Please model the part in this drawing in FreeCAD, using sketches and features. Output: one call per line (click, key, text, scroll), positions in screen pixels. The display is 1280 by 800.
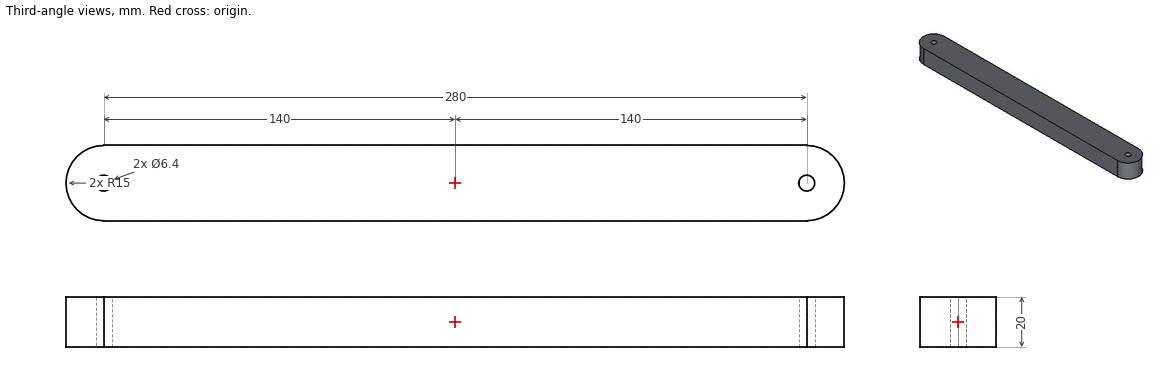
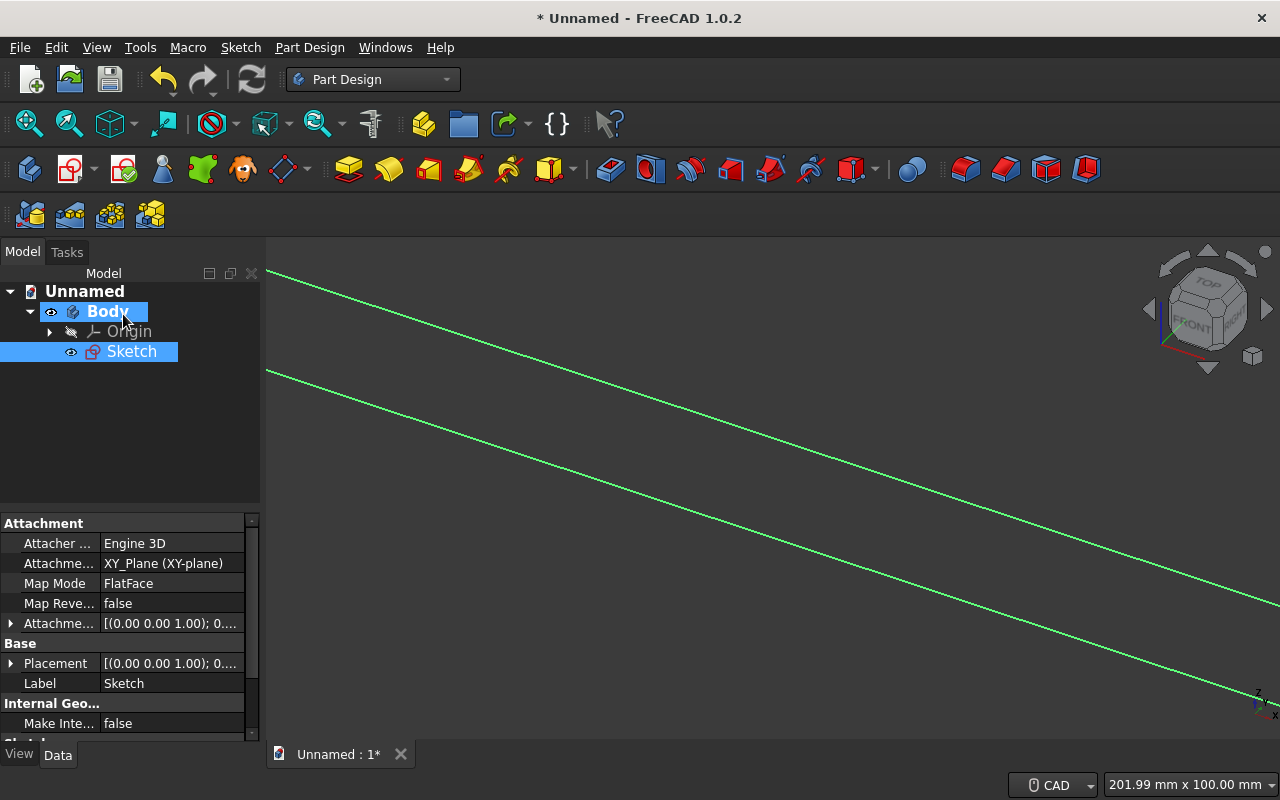
click(350, 170)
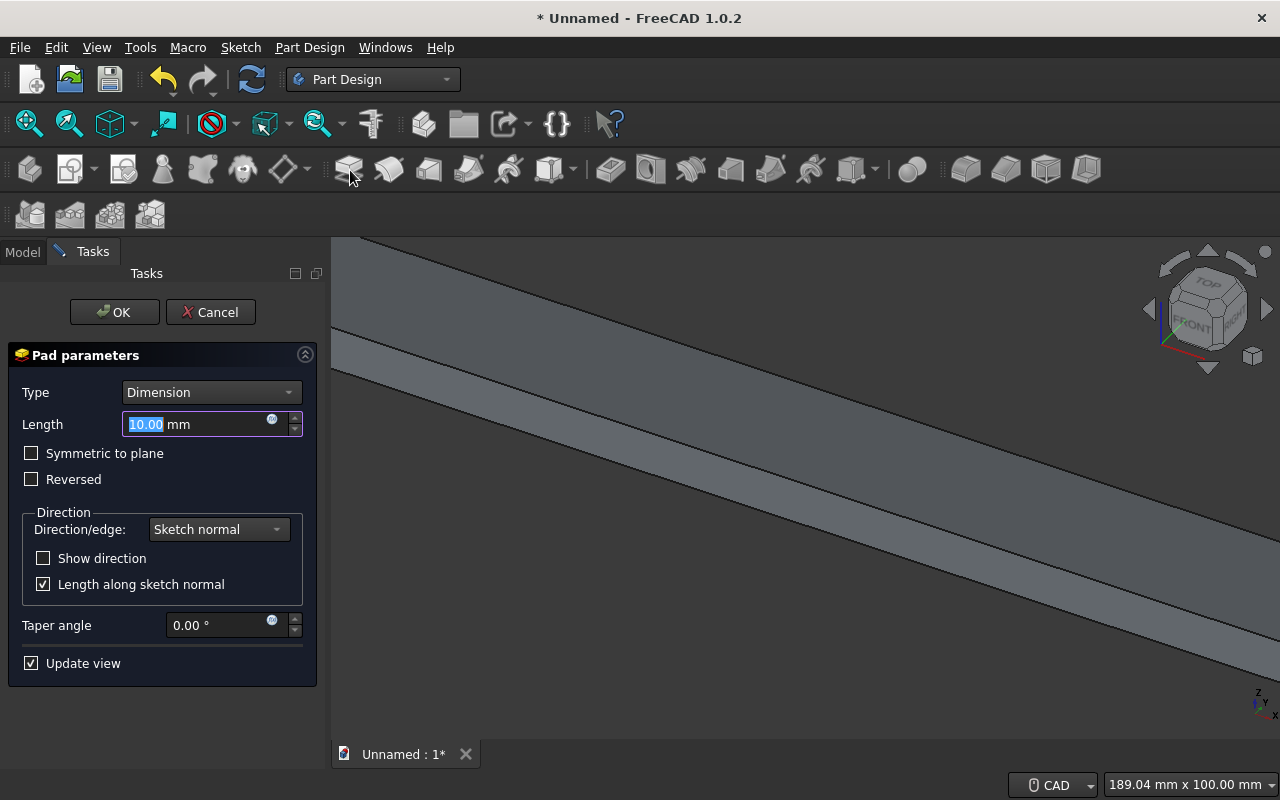
text(20)
key(Tab)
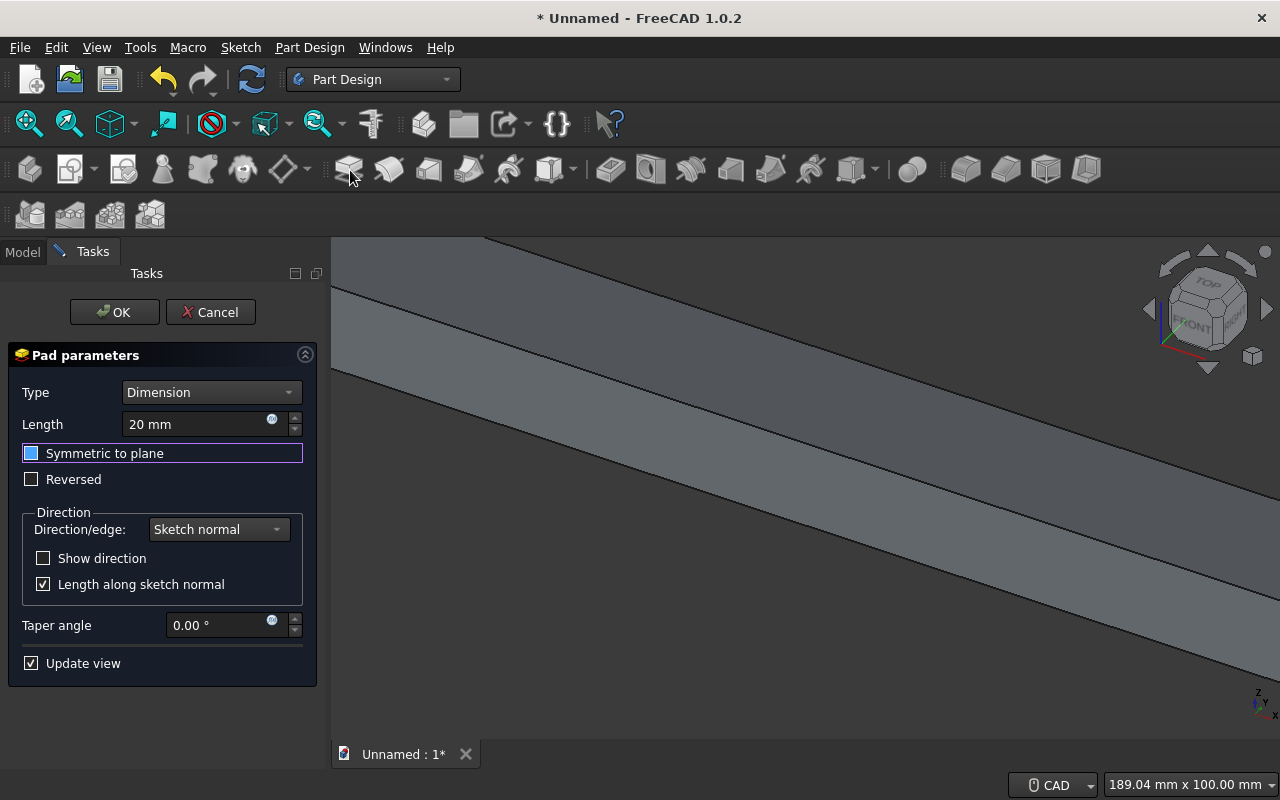
click(30, 453)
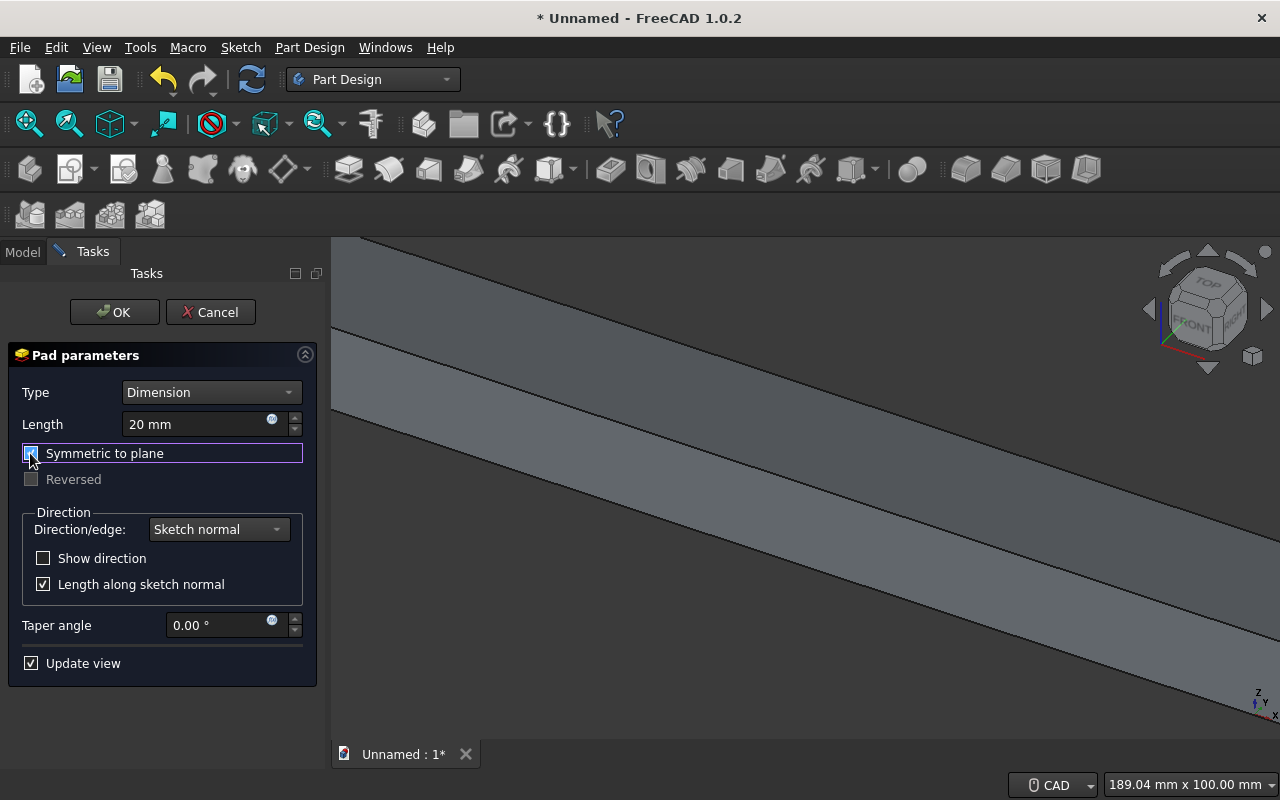
click(115, 312)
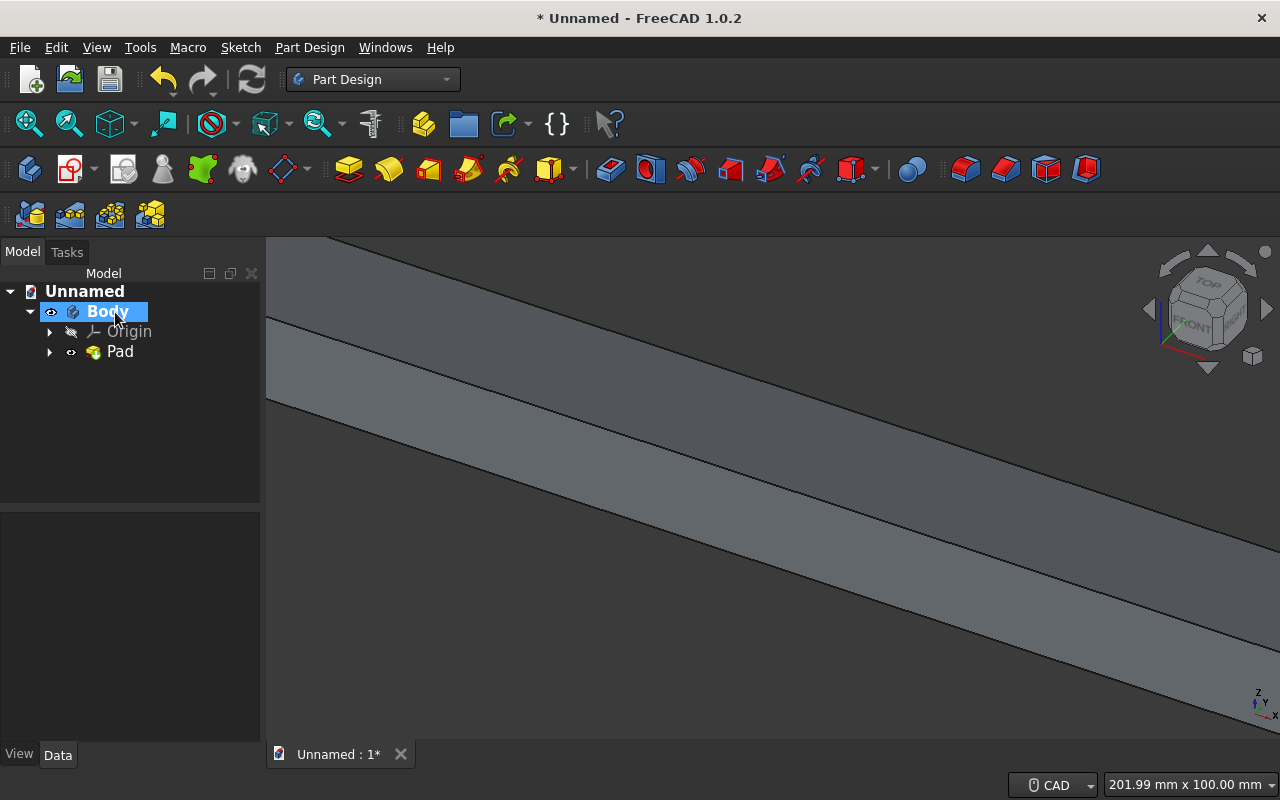
click(30, 124)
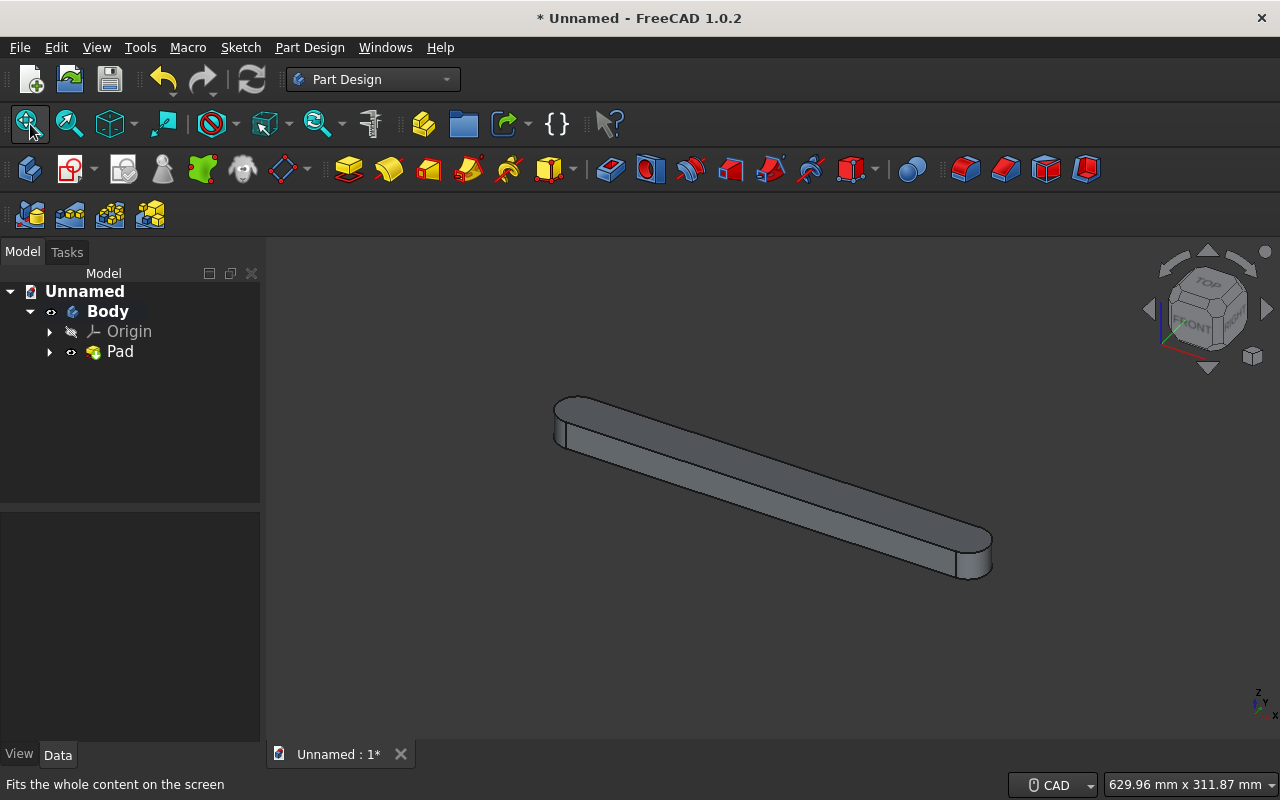
click(70, 170)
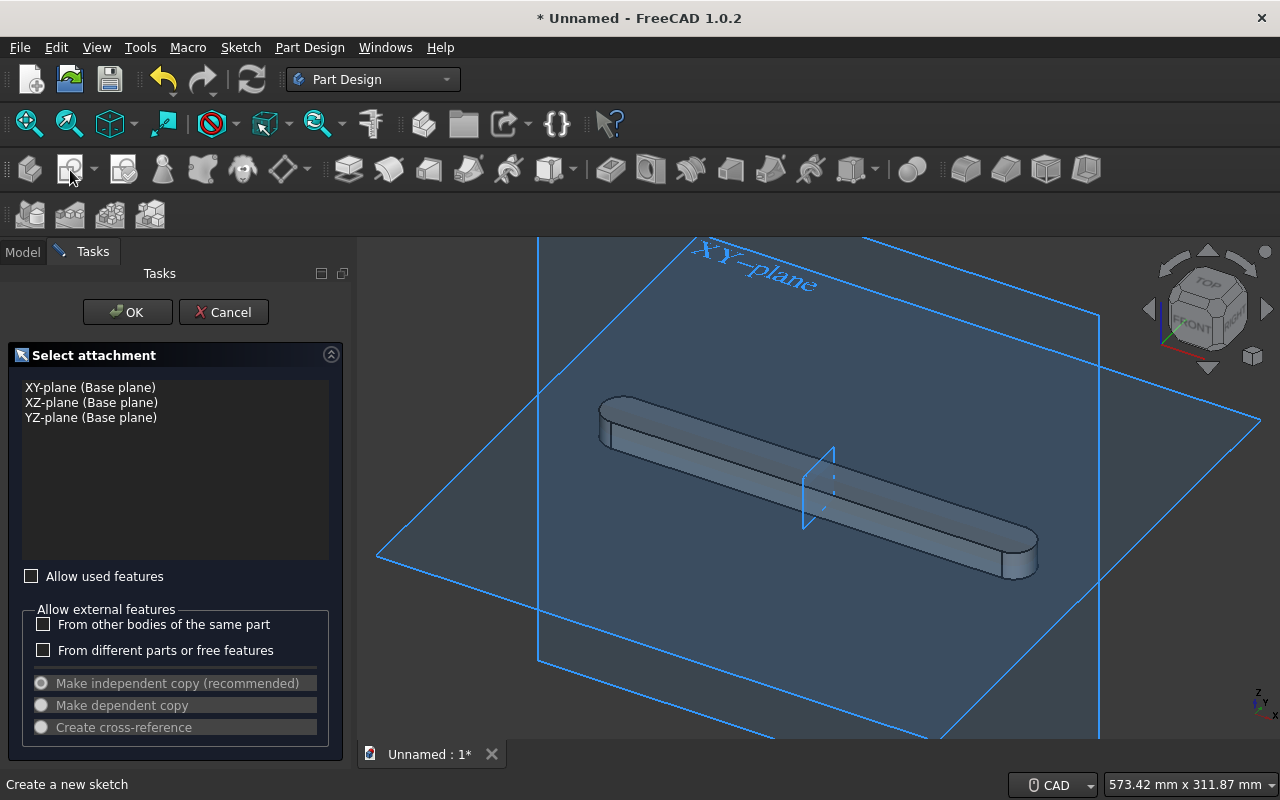
click(82, 388)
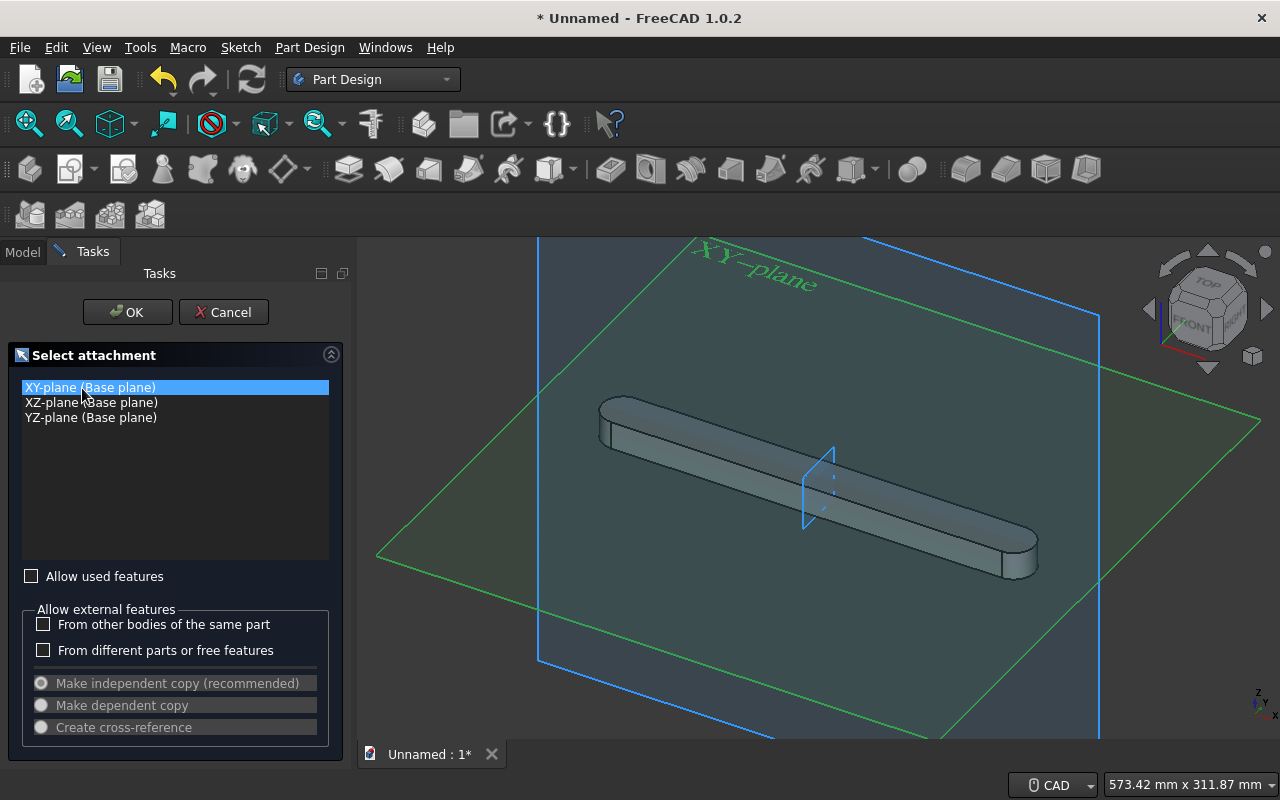
click(128, 312)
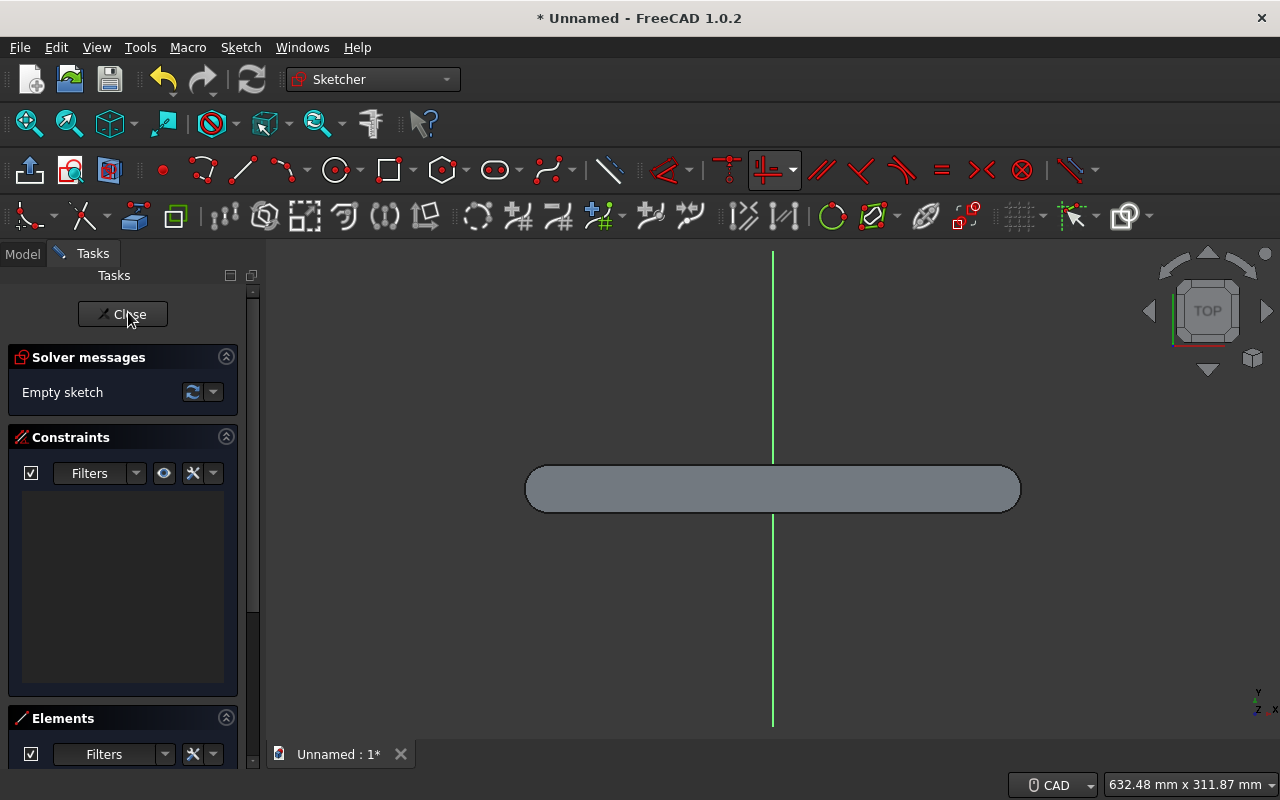
click(110, 170)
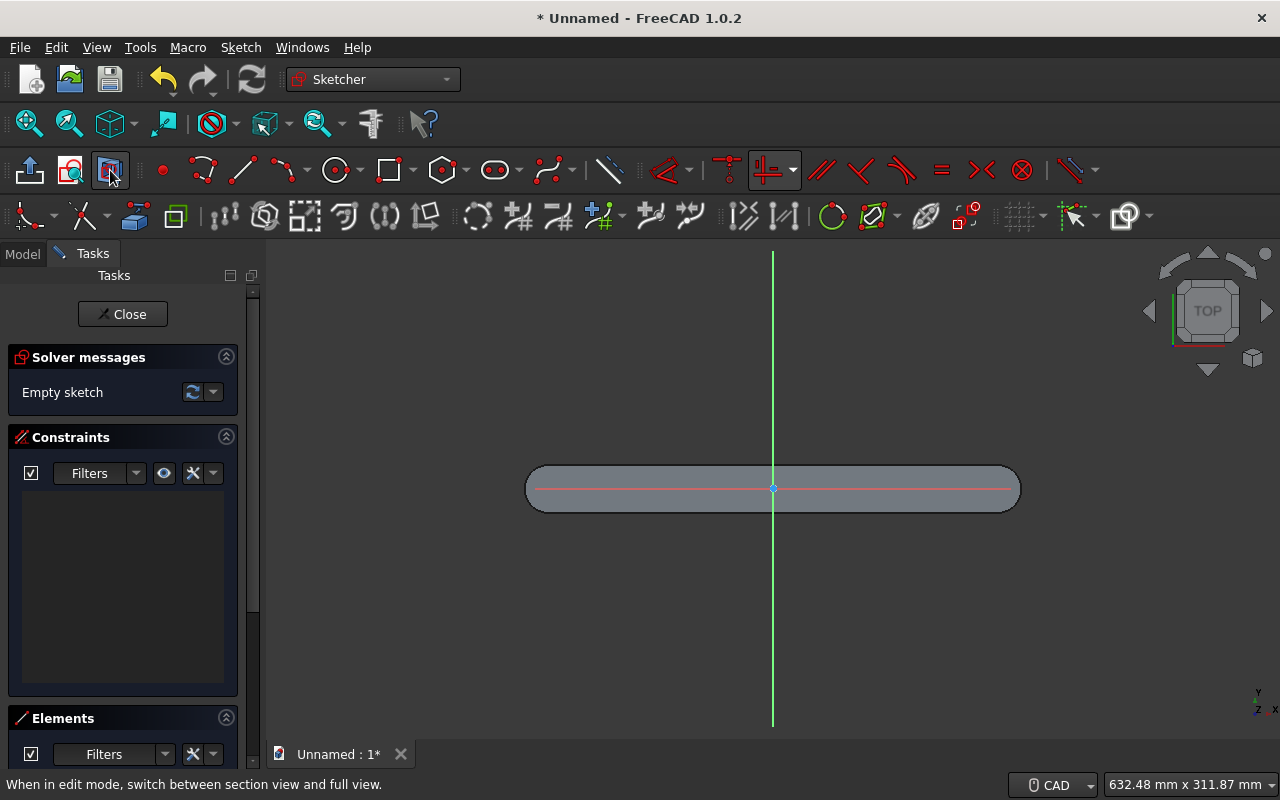
click(336, 170)